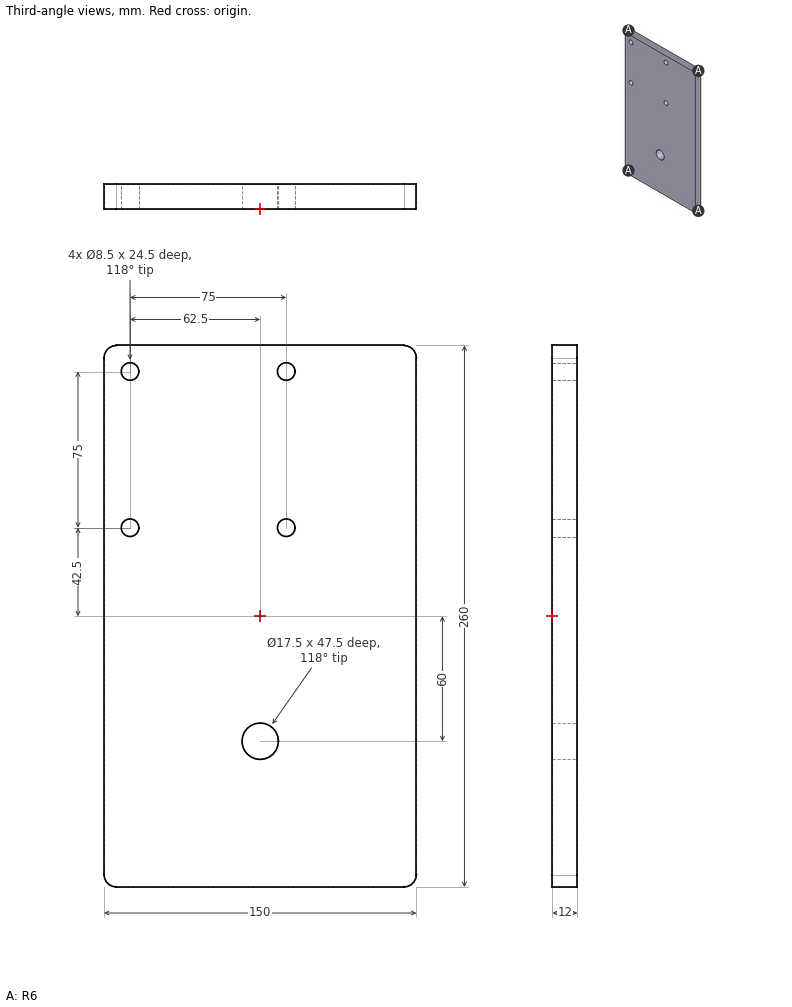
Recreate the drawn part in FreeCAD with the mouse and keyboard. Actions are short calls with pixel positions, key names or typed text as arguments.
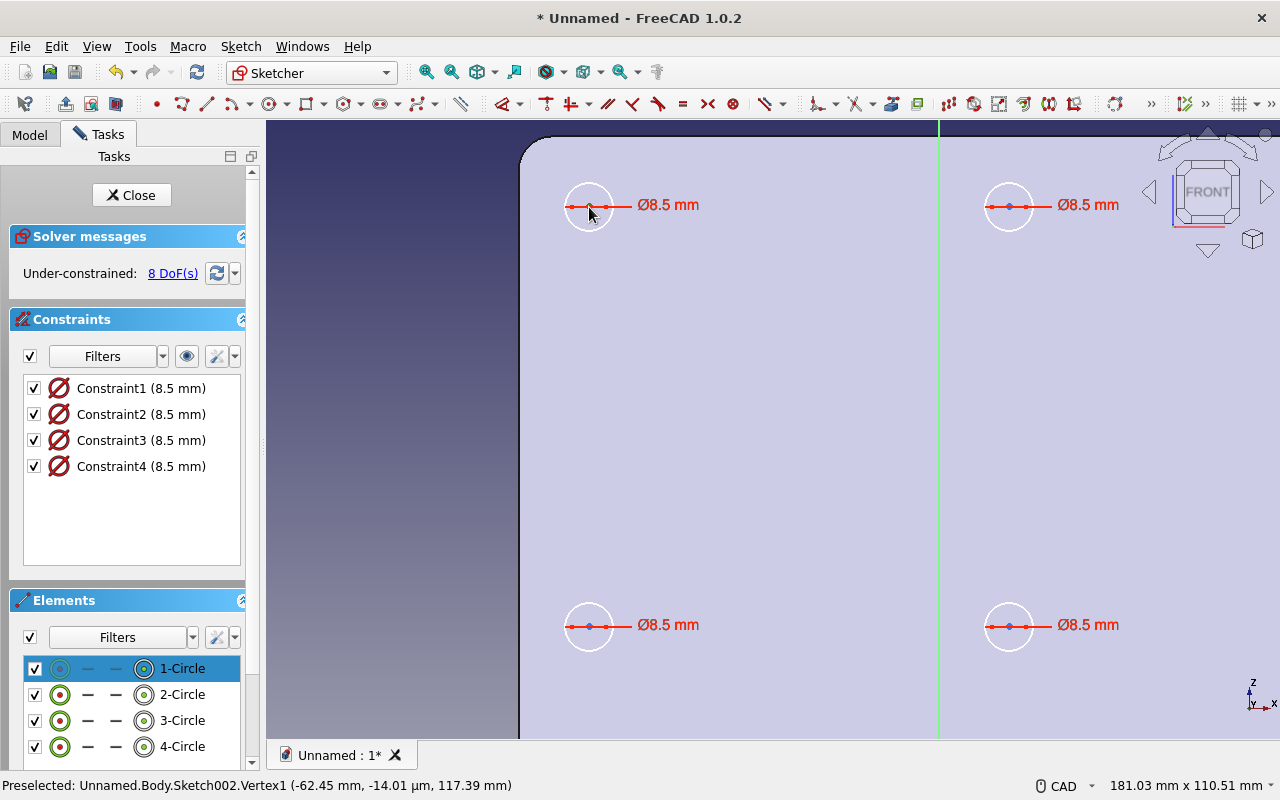
click(589, 627)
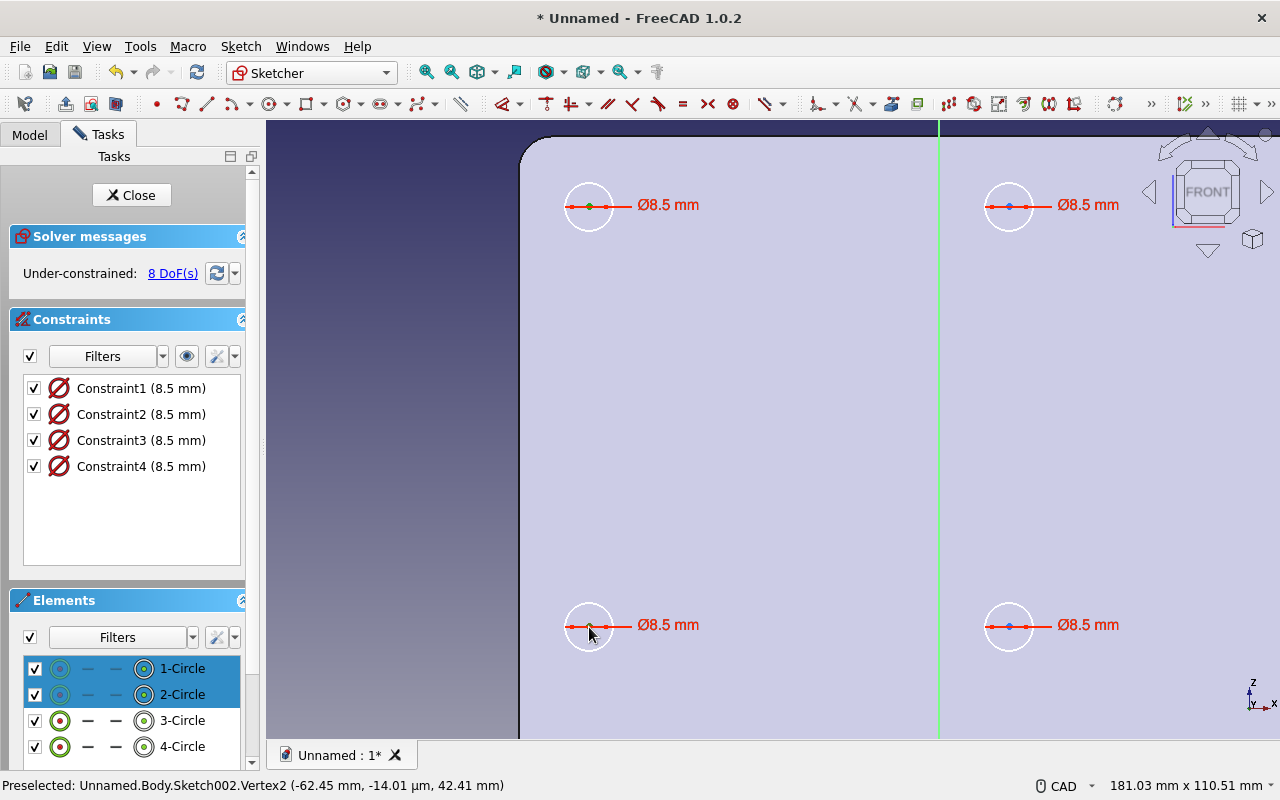
key(v)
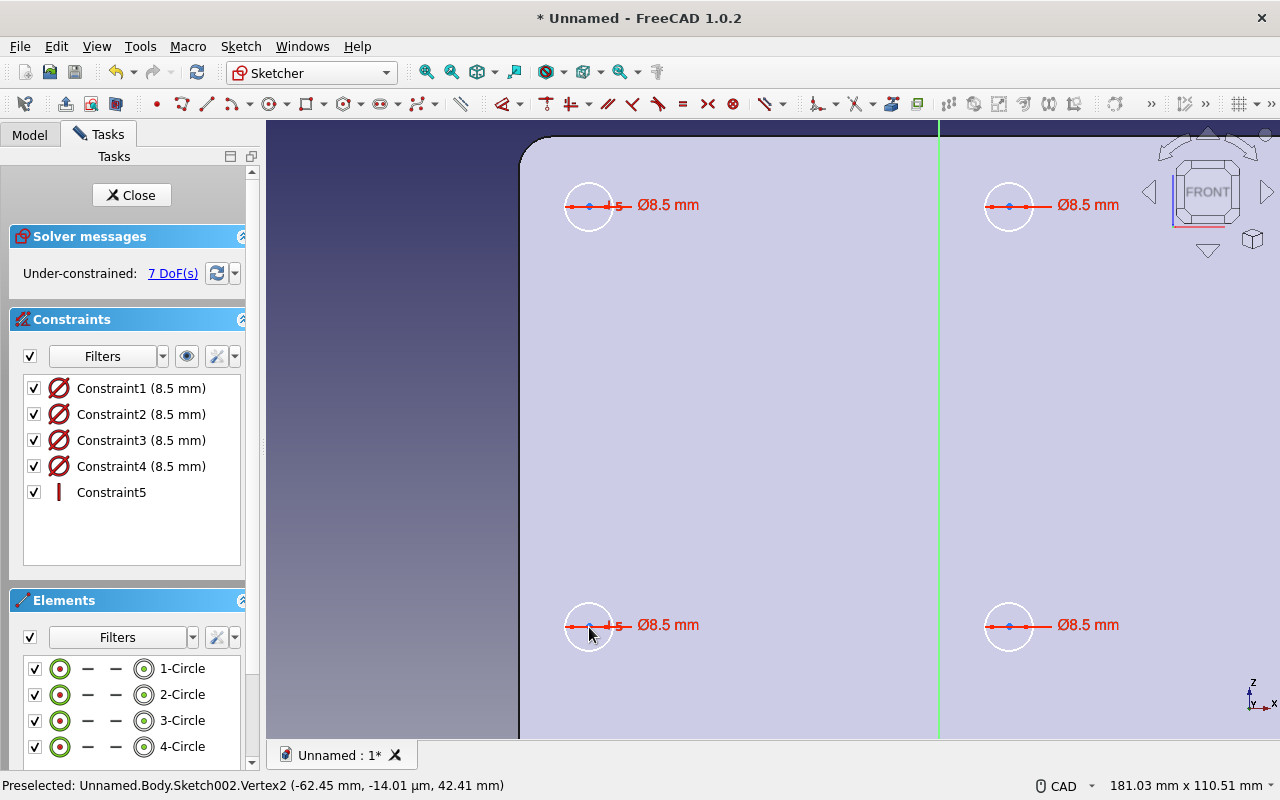
click(589, 627)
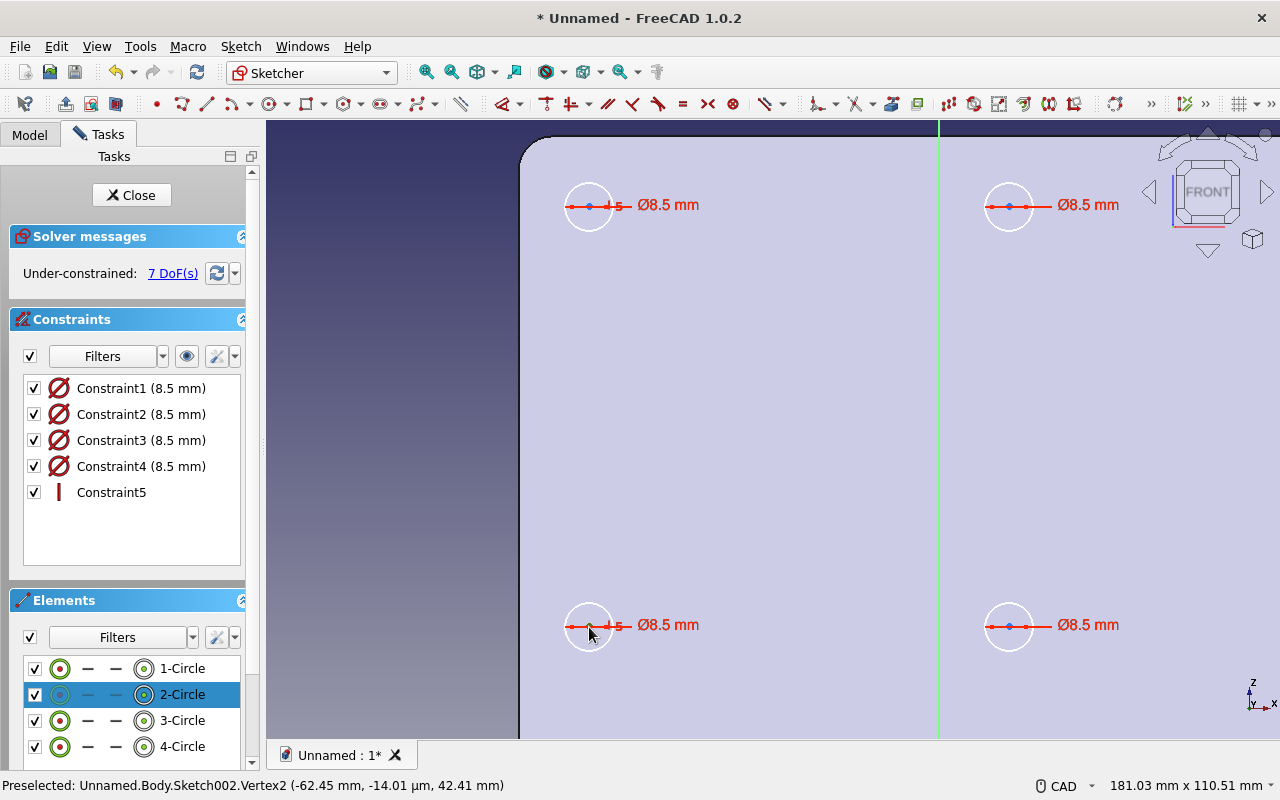
click(1009, 627)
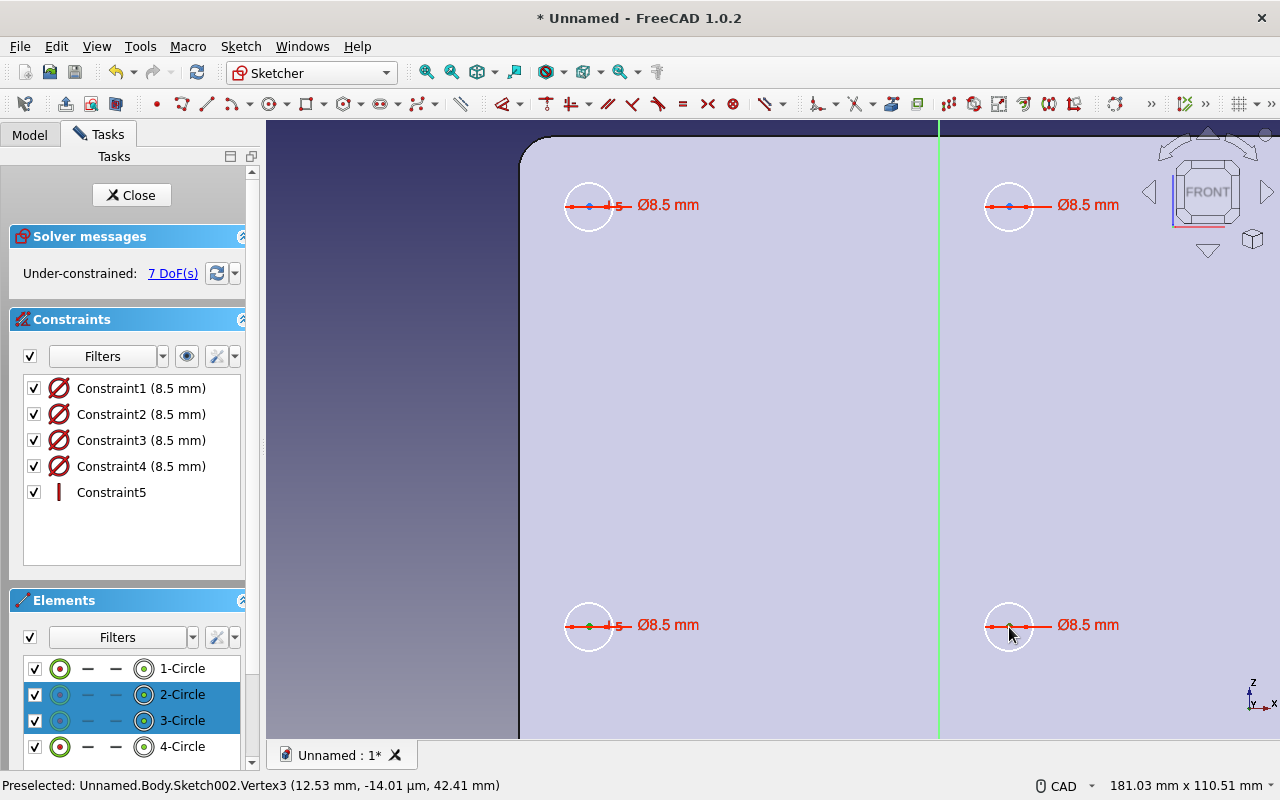
key(h)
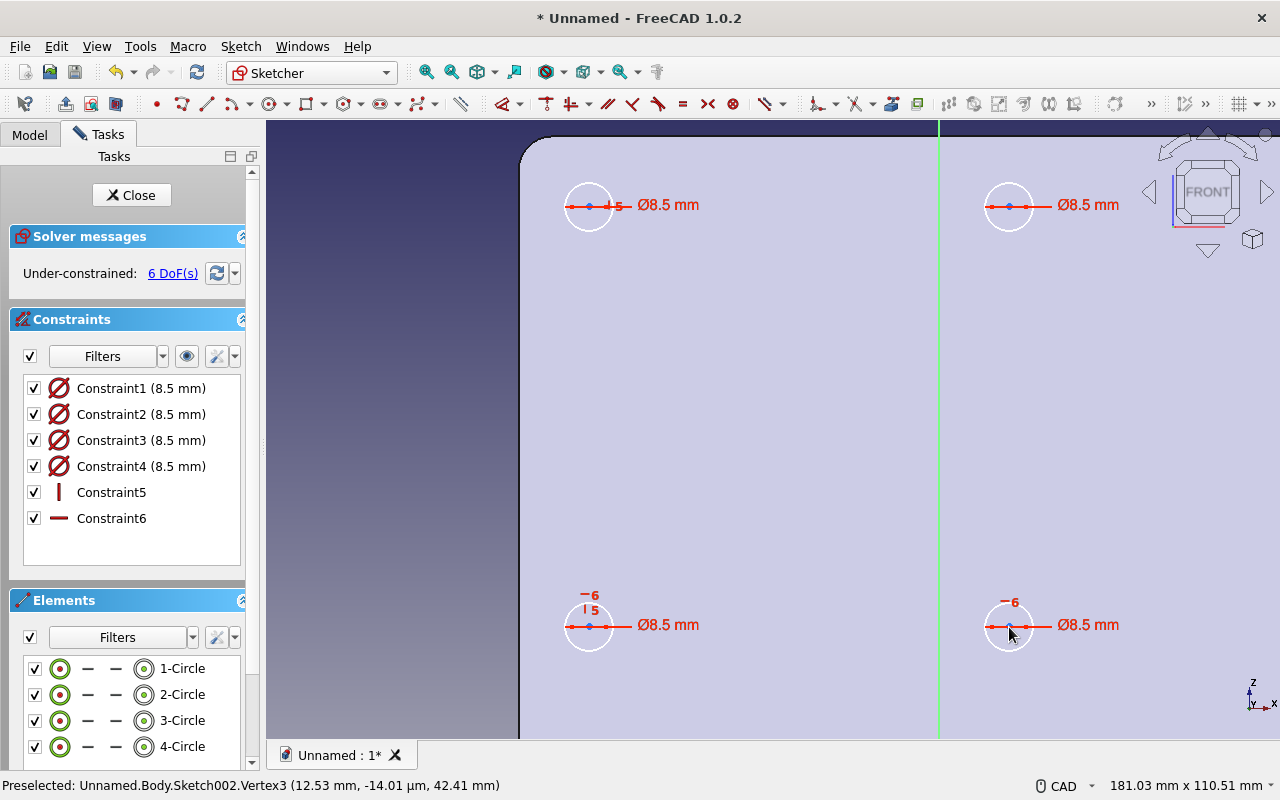
click(1009, 627)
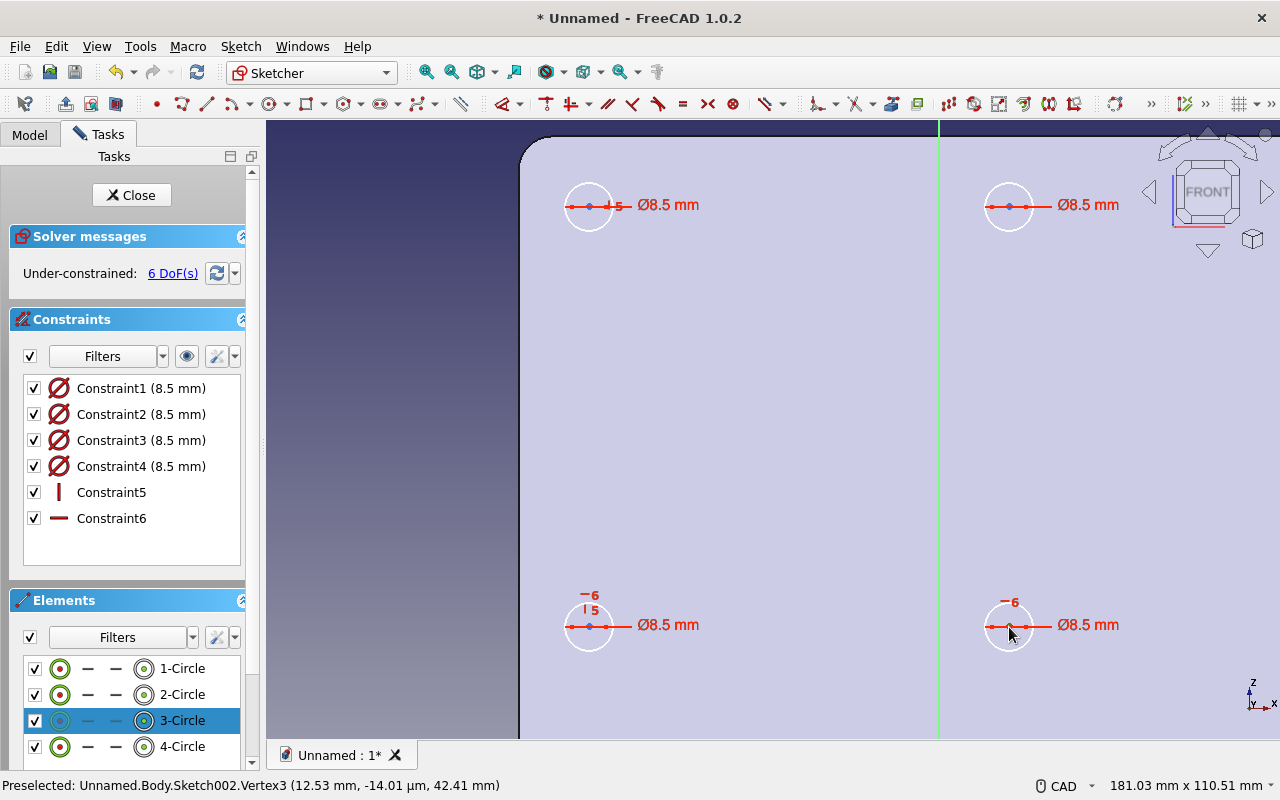
click(1009, 207)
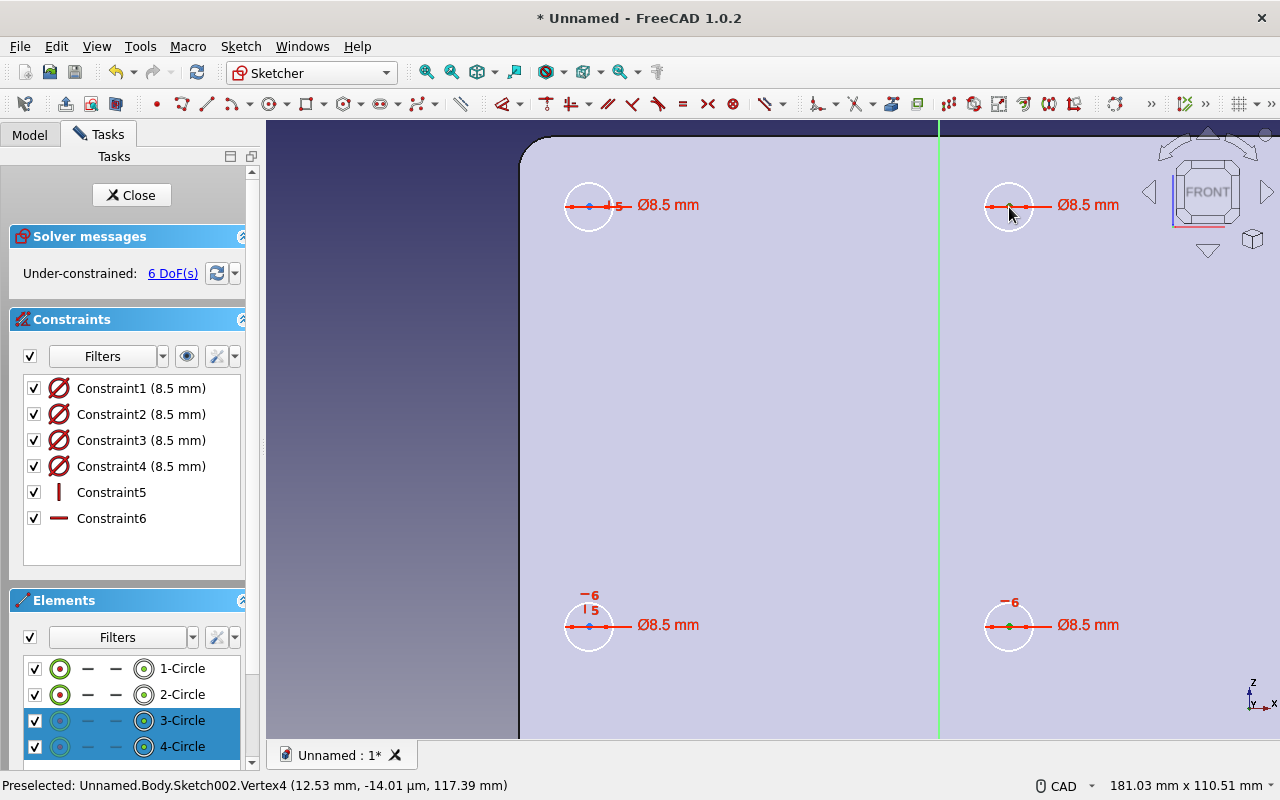
key(v)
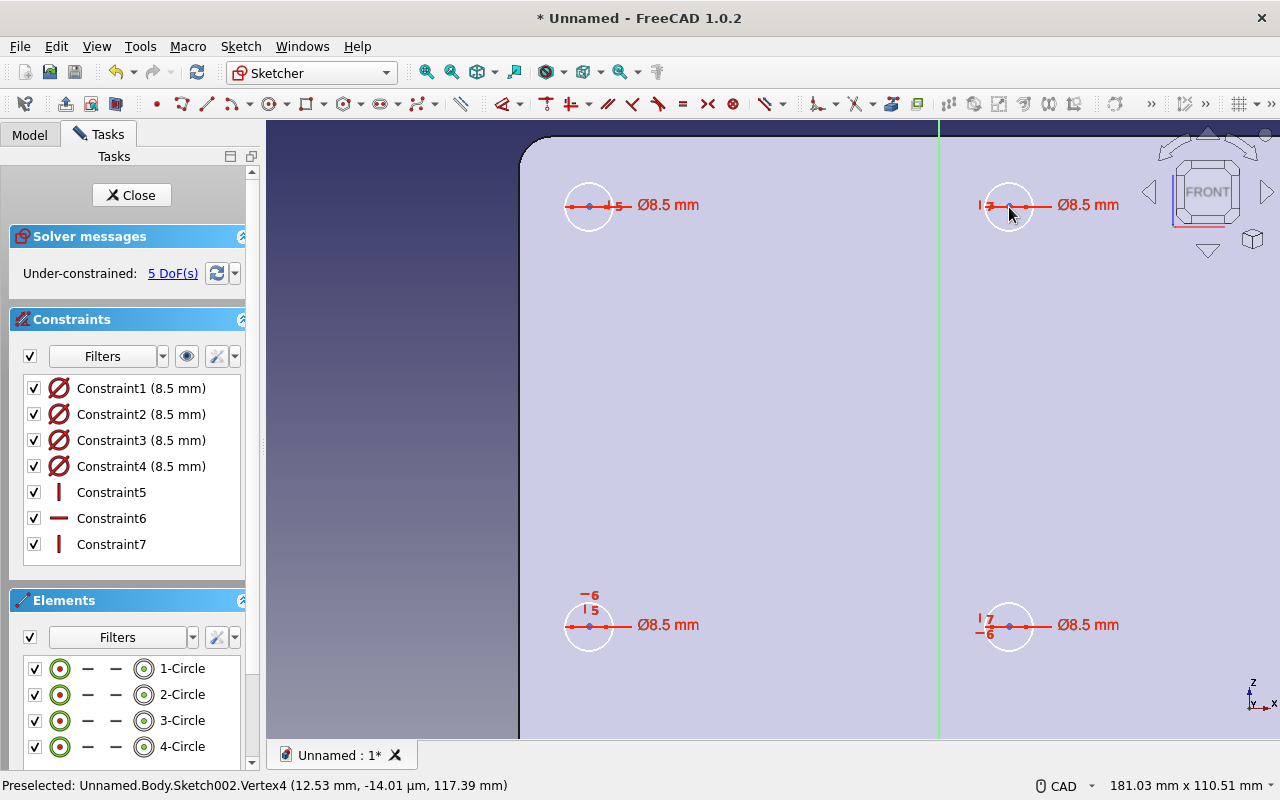
click(589, 207)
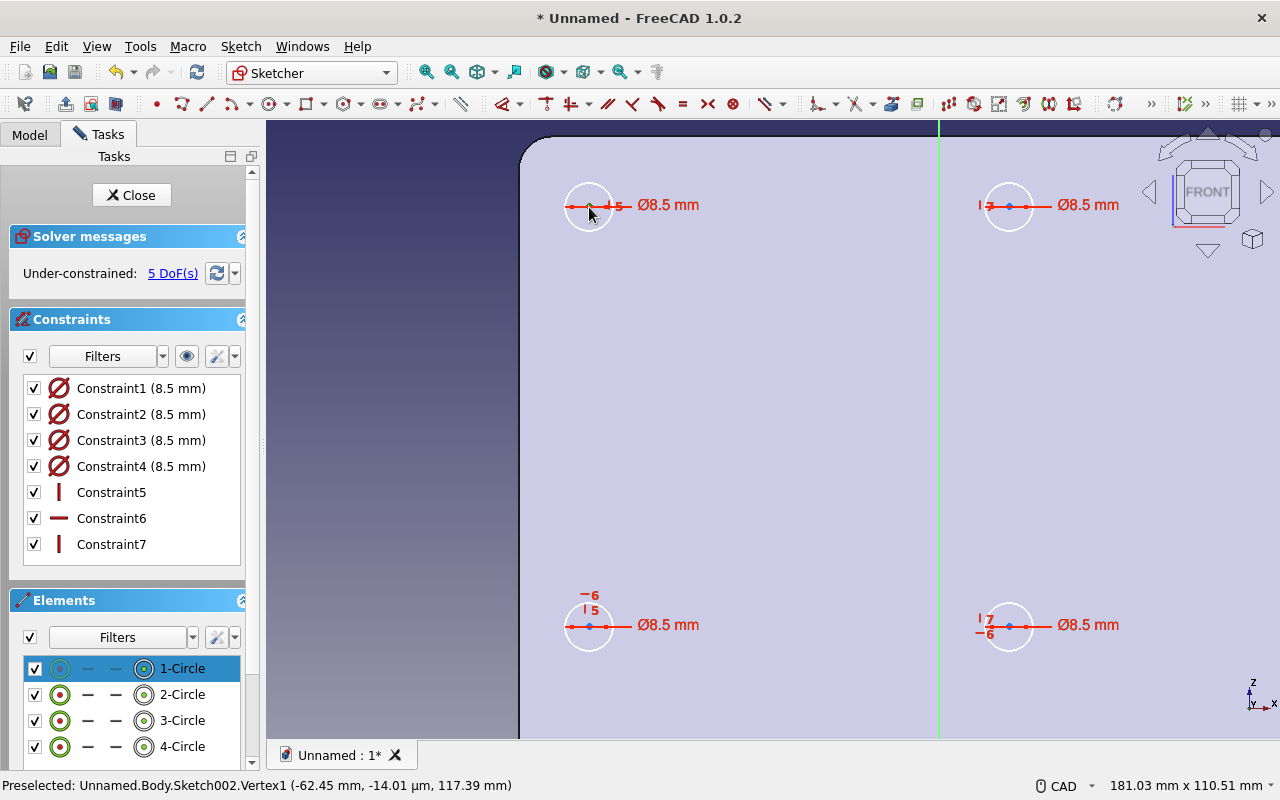
click(1009, 207)